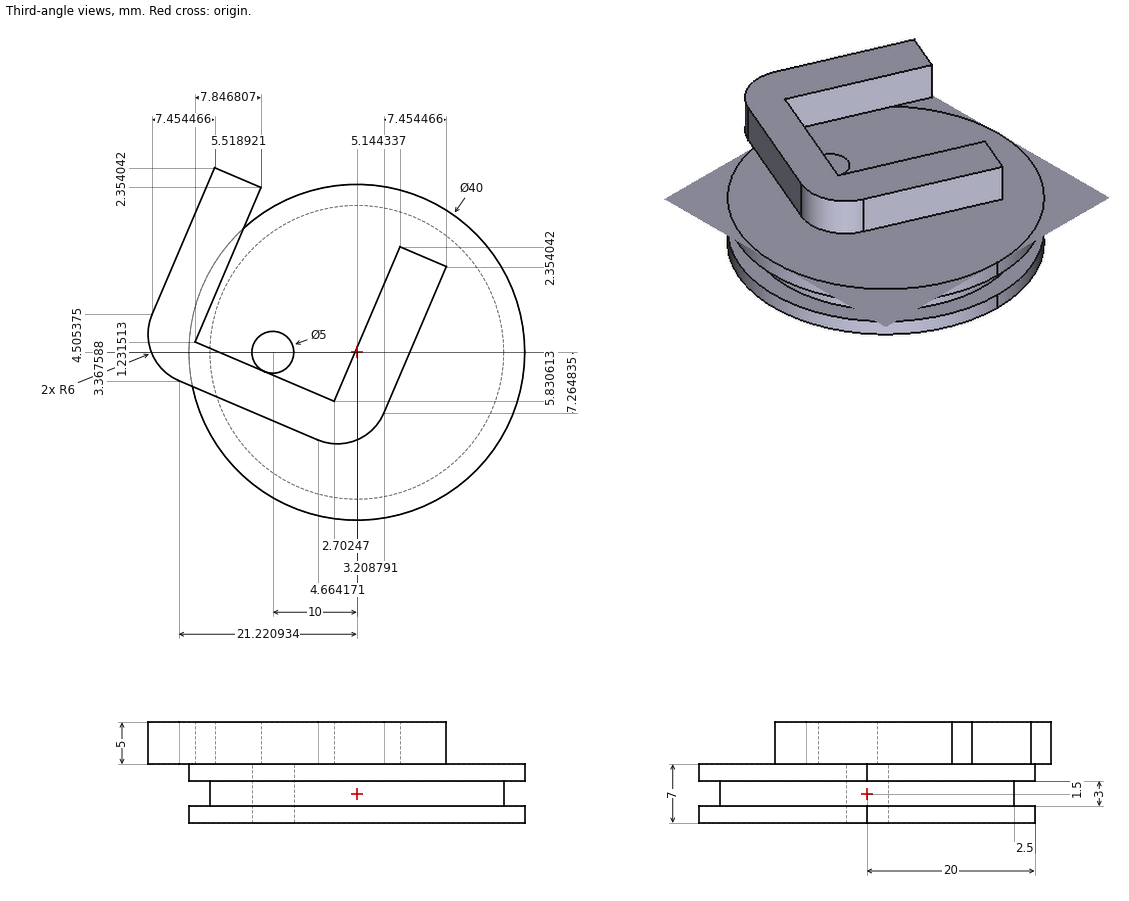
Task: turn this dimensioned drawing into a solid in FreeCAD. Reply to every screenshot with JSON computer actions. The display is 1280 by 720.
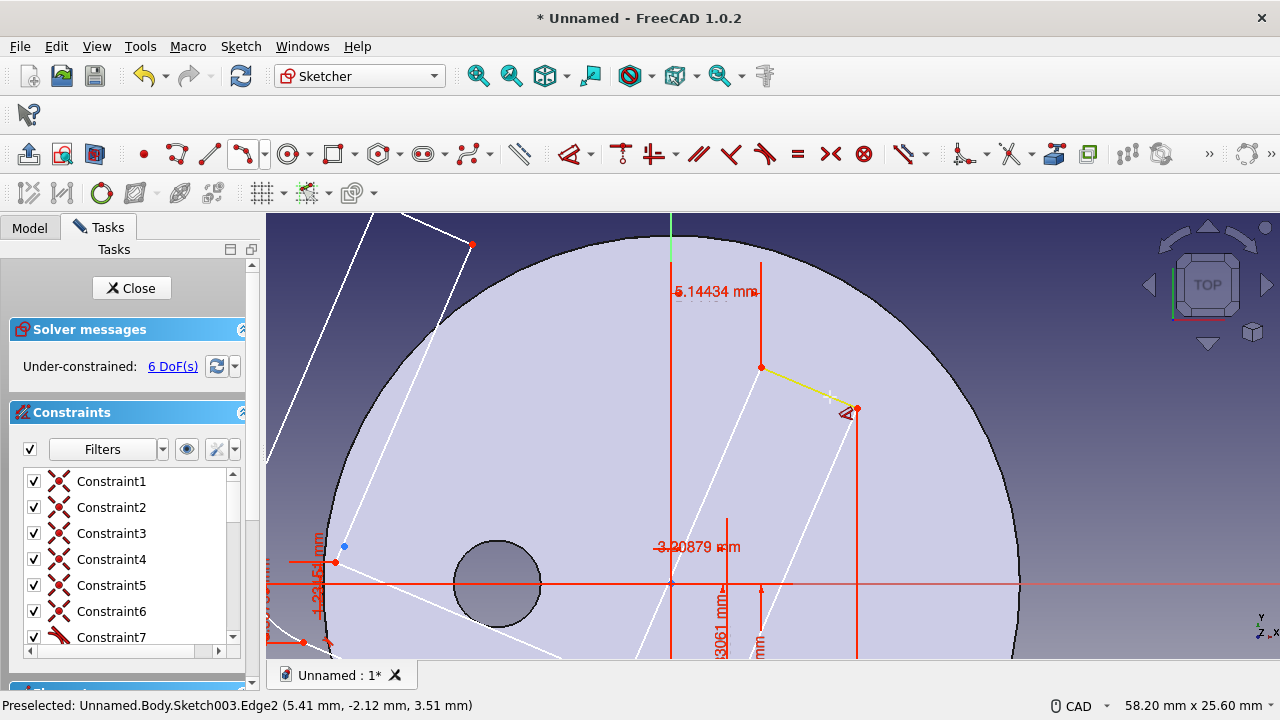
{"action": "left_click", "coordinate": [828, 396]}
{"action": "left_click", "coordinate": [891, 388]}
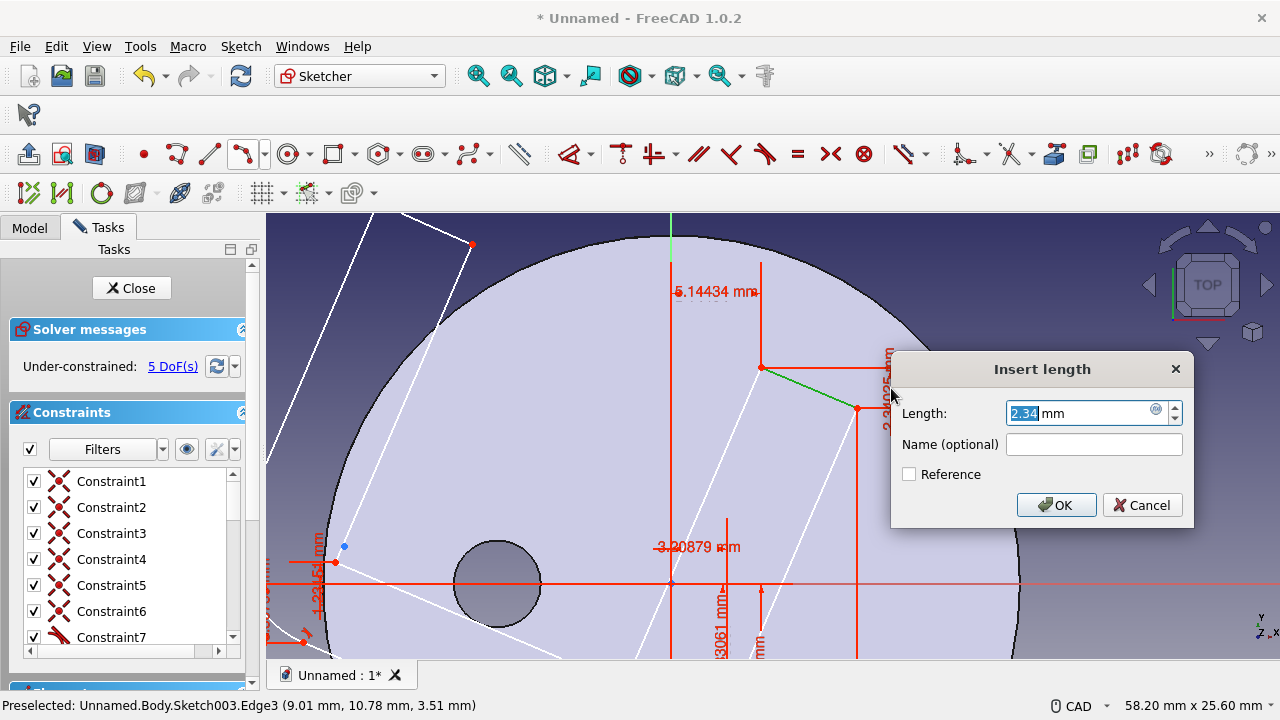
{"action": "type", "text": "2.354042"}
{"action": "key", "text": "Return"}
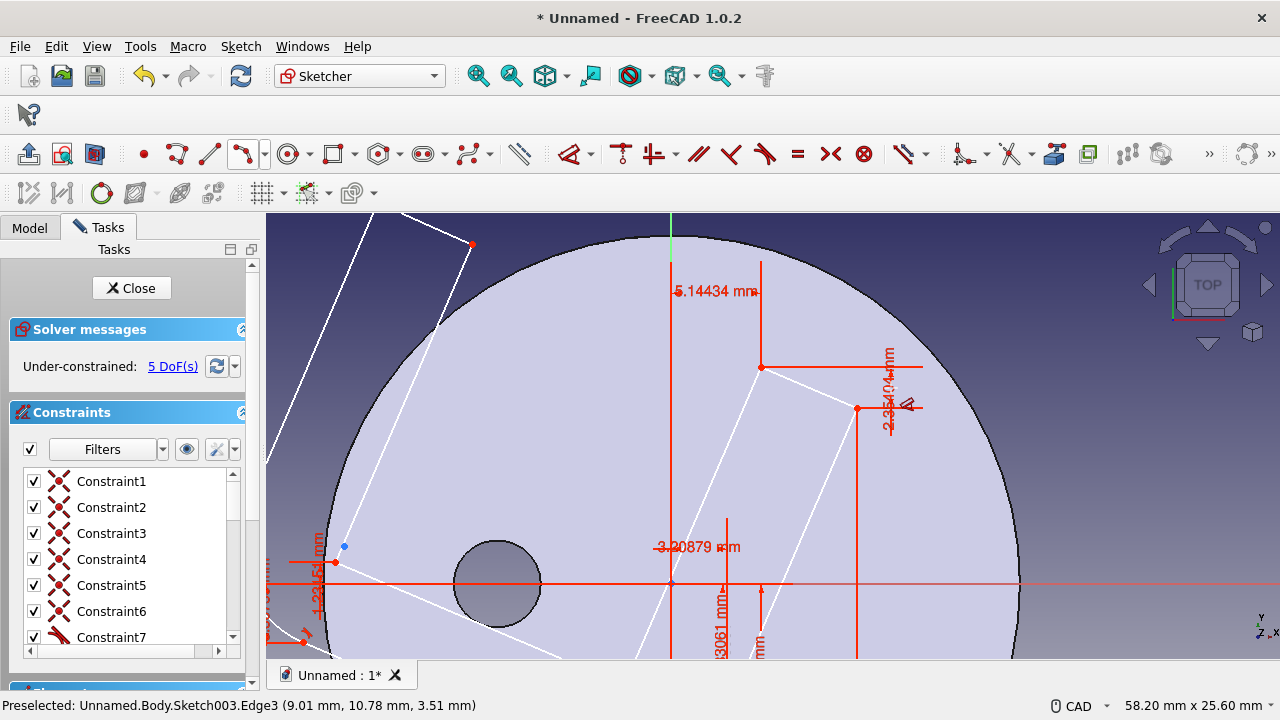
{"action": "left_click", "coordinate": [377, 467]}
{"action": "left_click", "coordinate": [404, 620]}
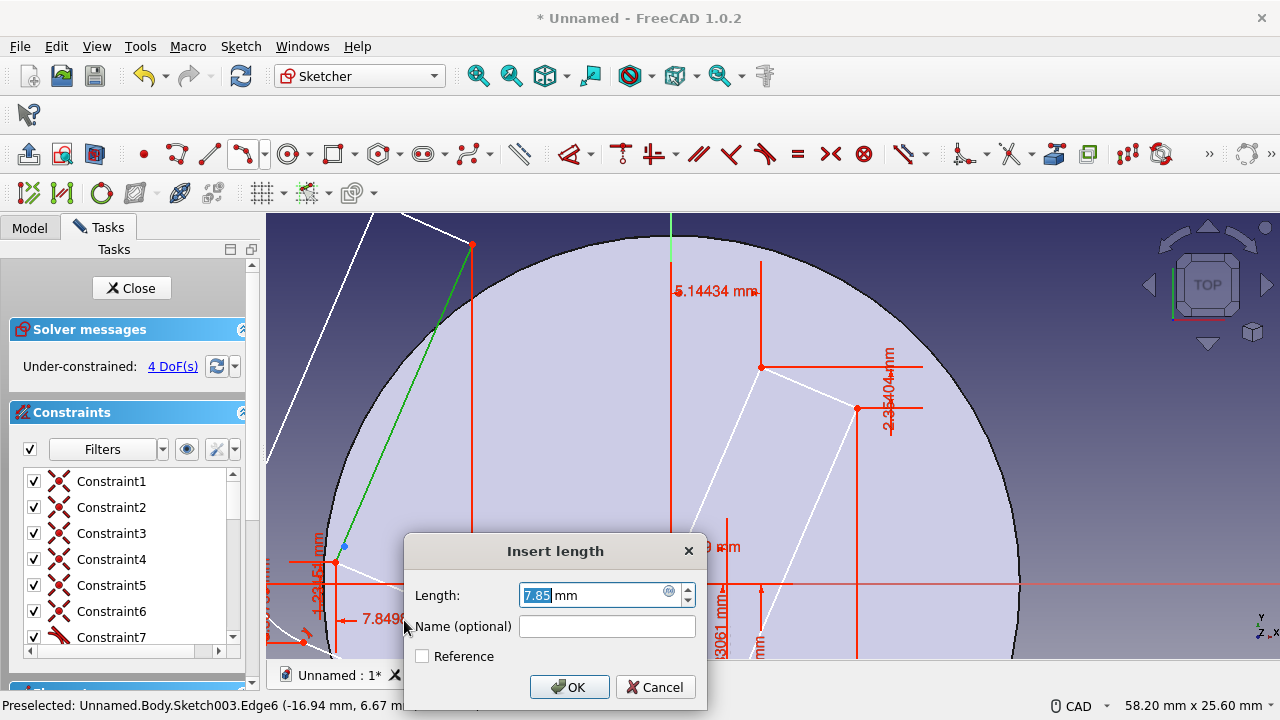
{"action": "type", "text": "7.846807"}
{"action": "key", "text": "Return"}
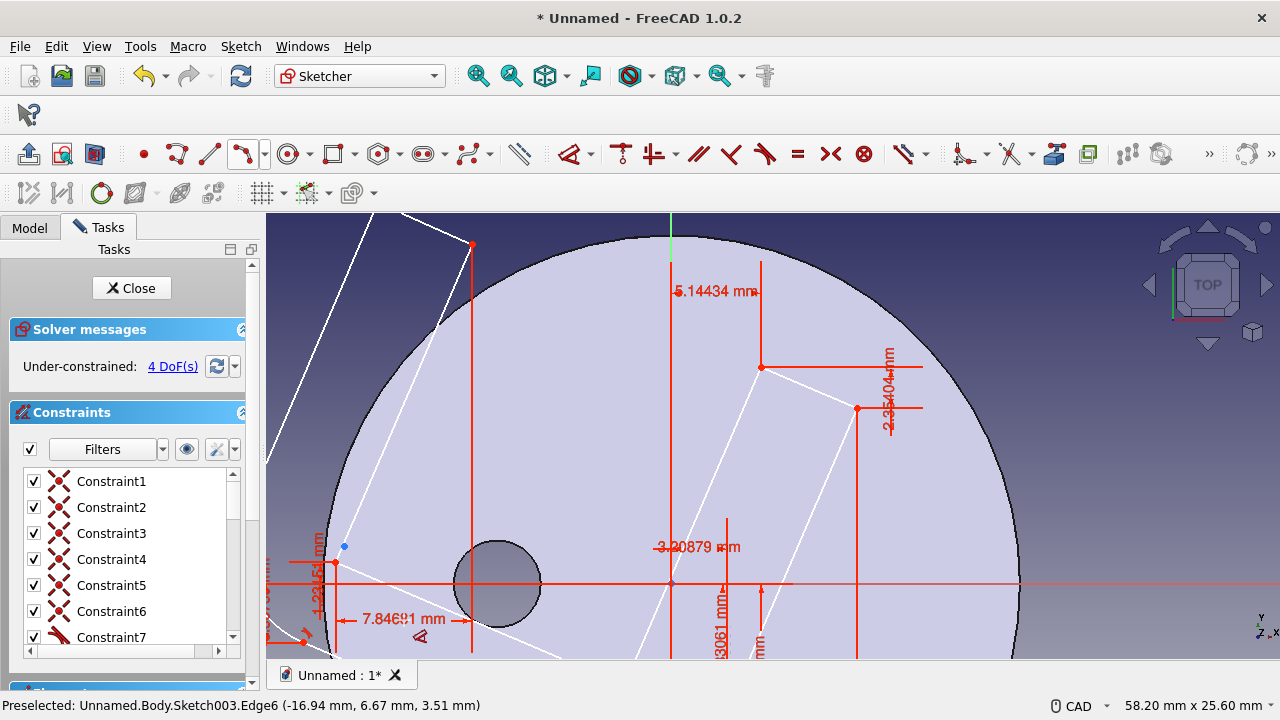
{"action": "scroll", "coordinate": [829, 397], "scroll_direction": "down", "scroll_amount": 4}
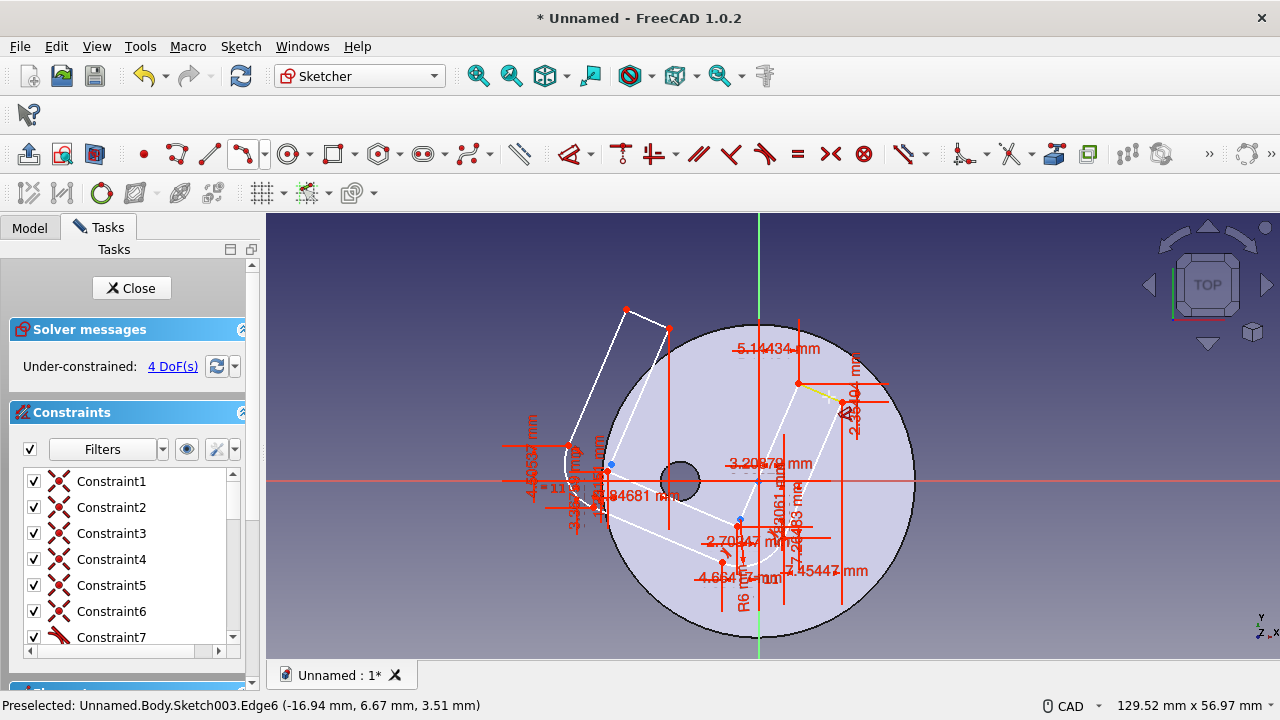
{"action": "left_click", "coordinate": [656, 323]}
{"action": "left_click", "coordinate": [648, 276]}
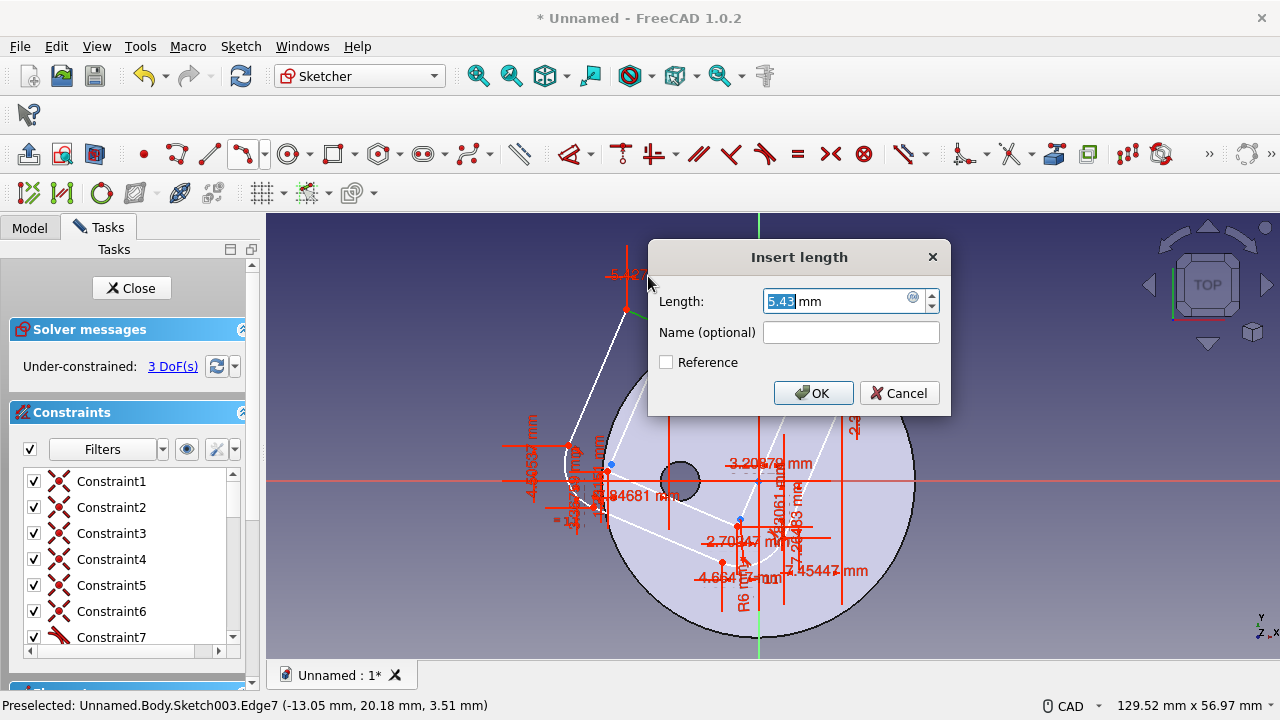
{"action": "type", "text": "5.518921"}
{"action": "key", "text": "Return"}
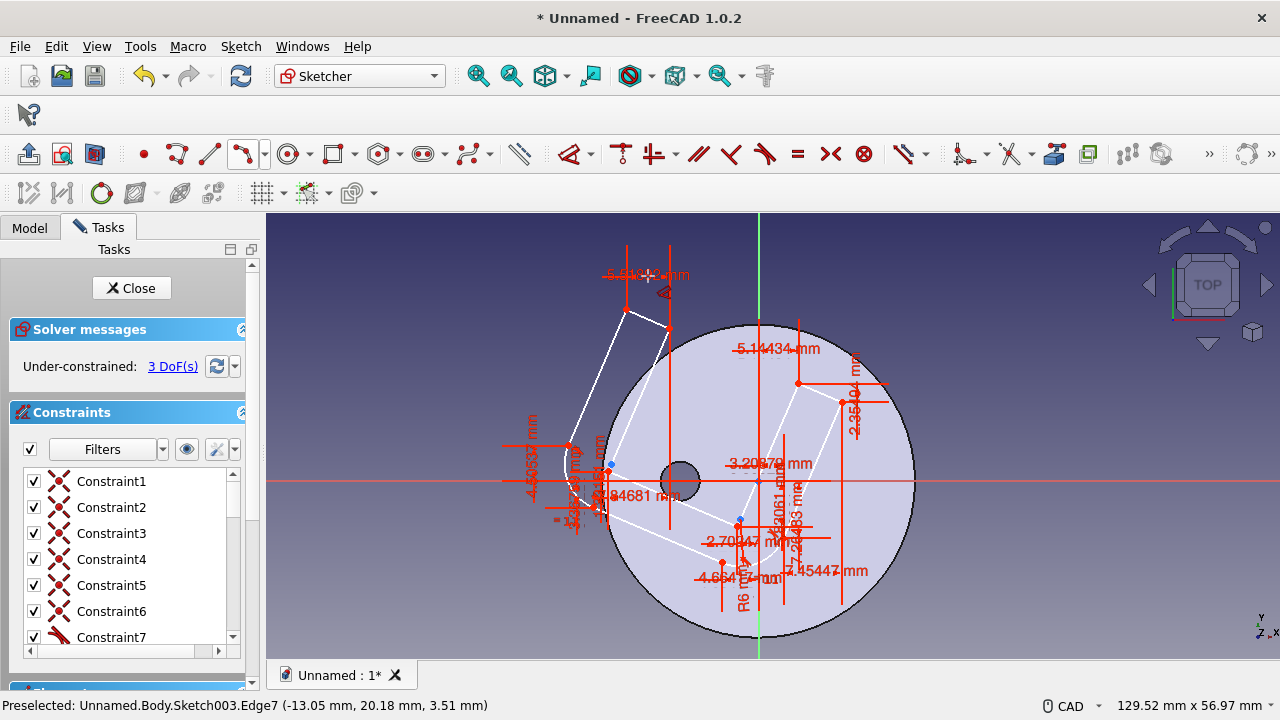
{"action": "scroll", "coordinate": [657, 323], "scroll_direction": "up", "scroll_amount": 4}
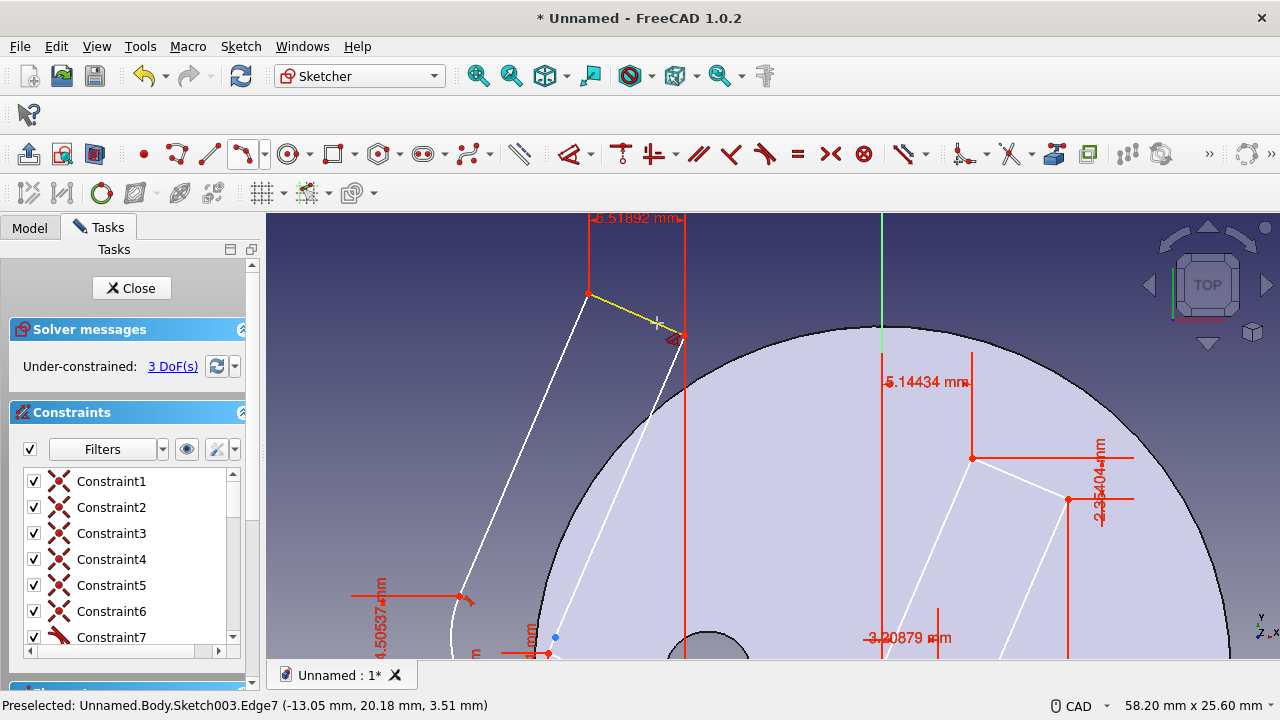
{"action": "left_click", "coordinate": [656, 323]}
{"action": "left_click", "coordinate": [555, 315]}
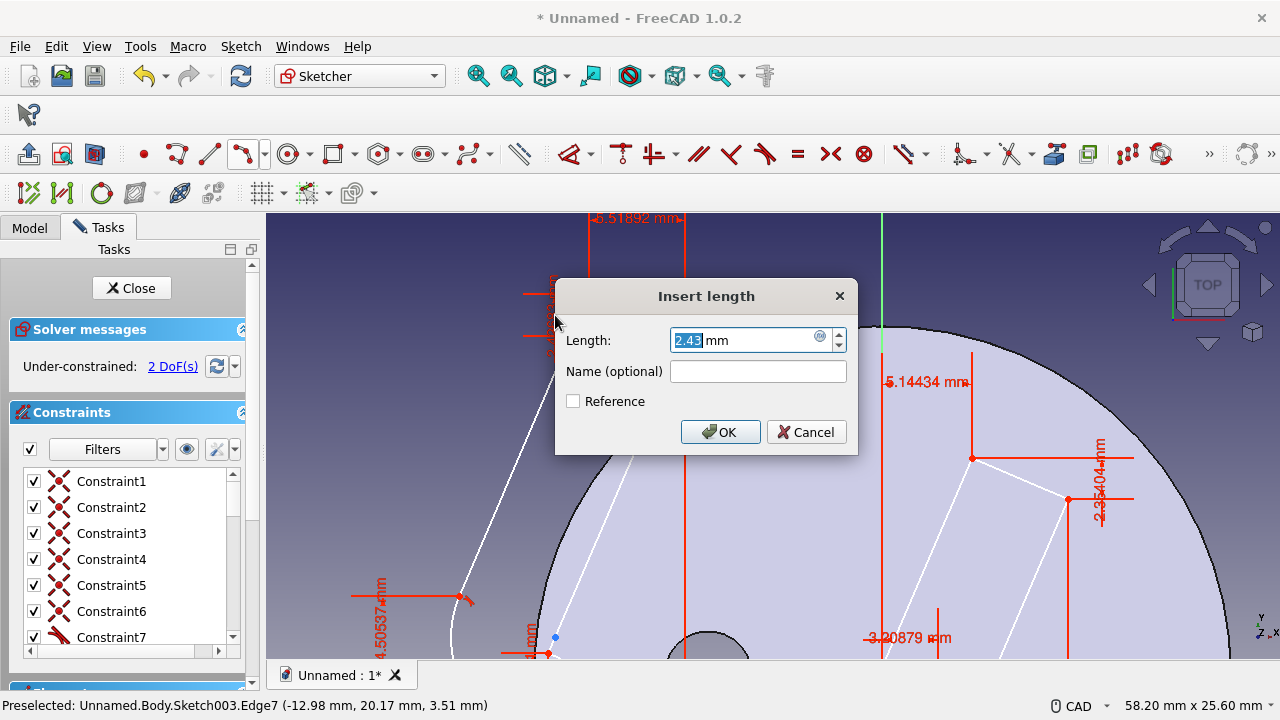
{"action": "type", "text": "2.354042"}
{"action": "key", "text": "Return"}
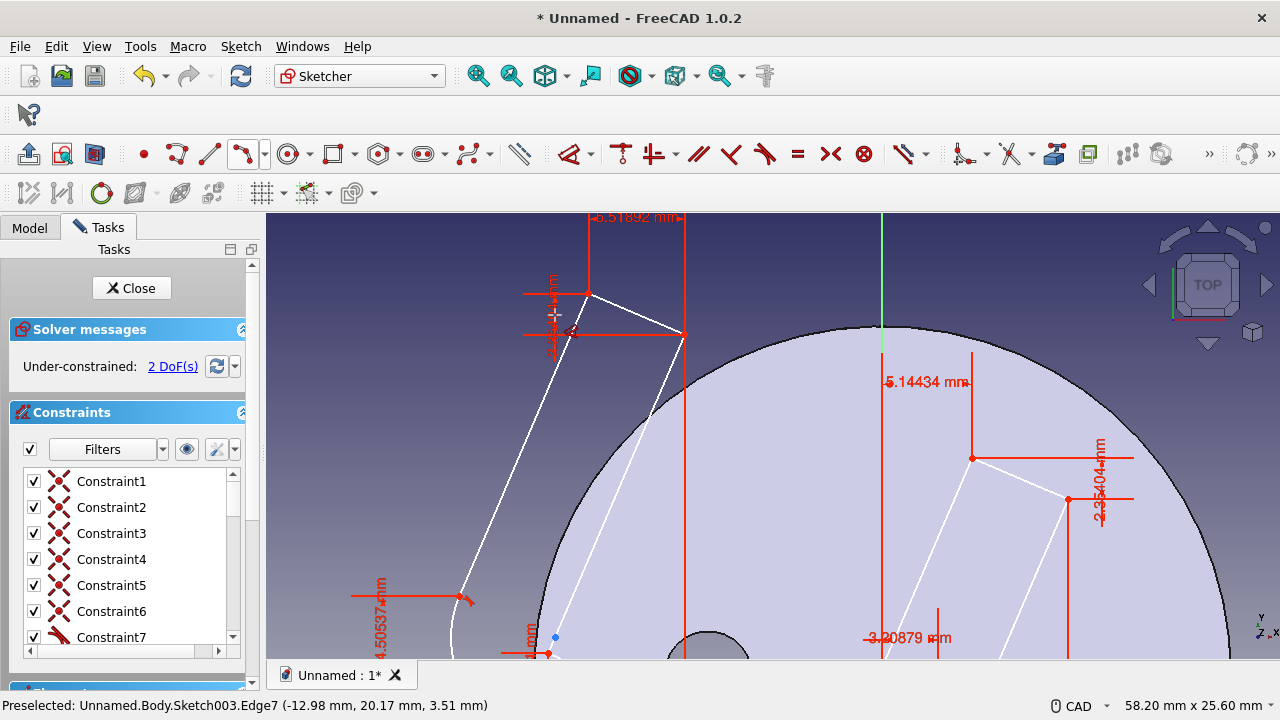
{"action": "left_click", "coordinate": [550, 384]}
{"action": "left_click", "coordinate": [524, 260]}